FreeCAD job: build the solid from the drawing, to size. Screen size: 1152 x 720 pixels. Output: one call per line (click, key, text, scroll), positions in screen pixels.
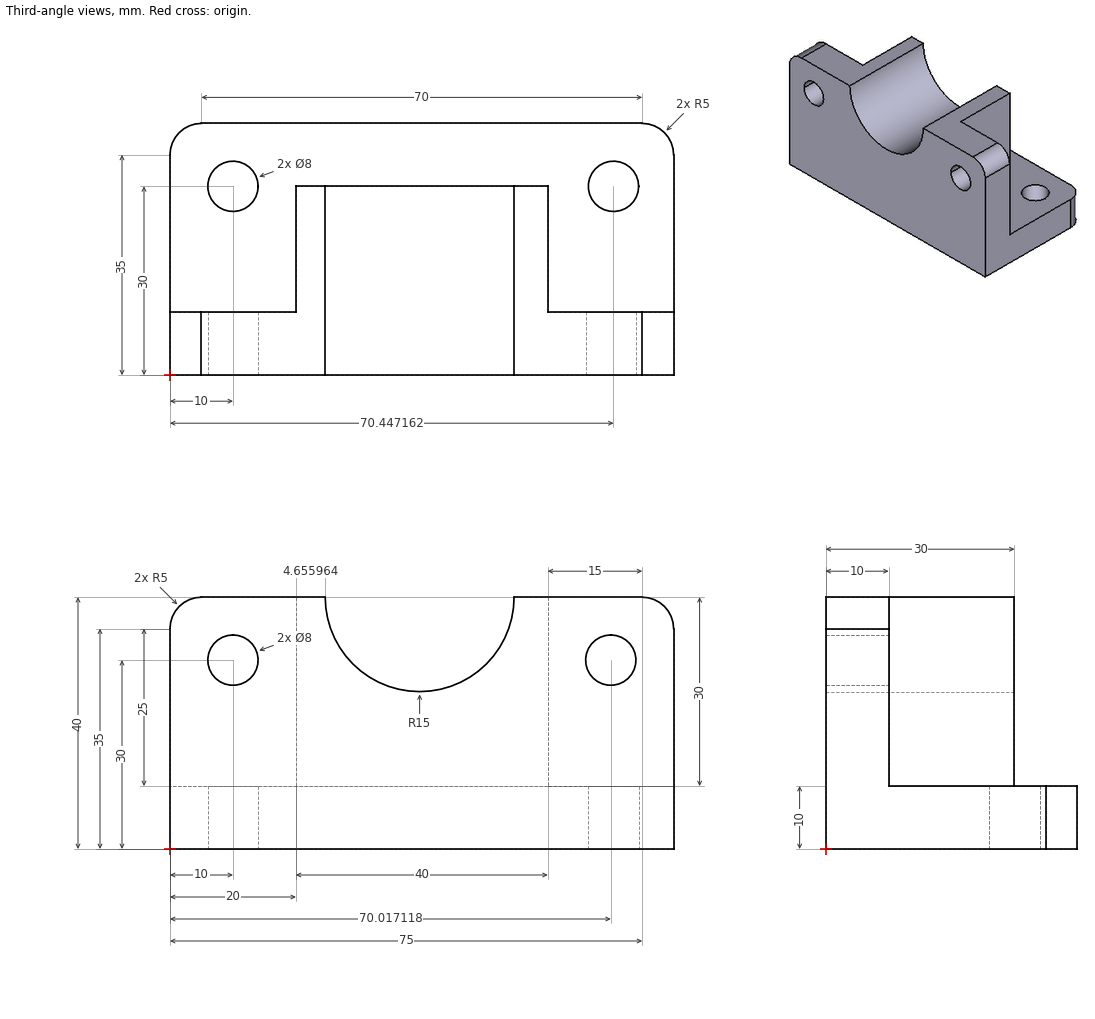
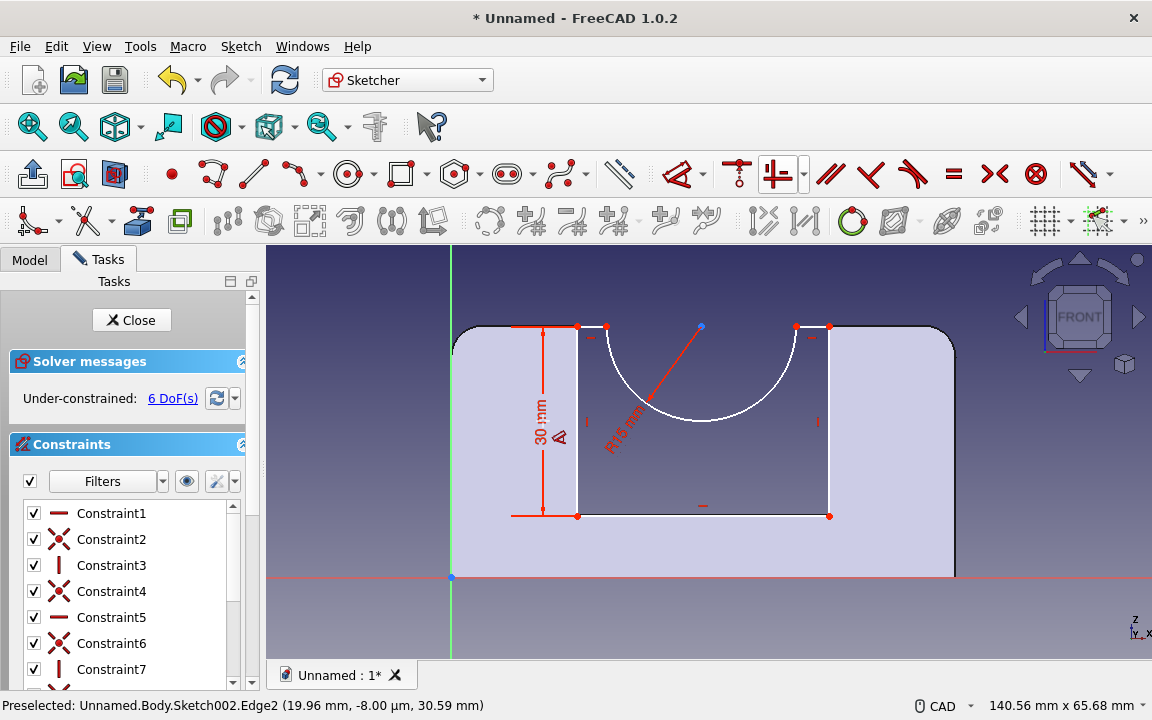
click(653, 516)
click(703, 550)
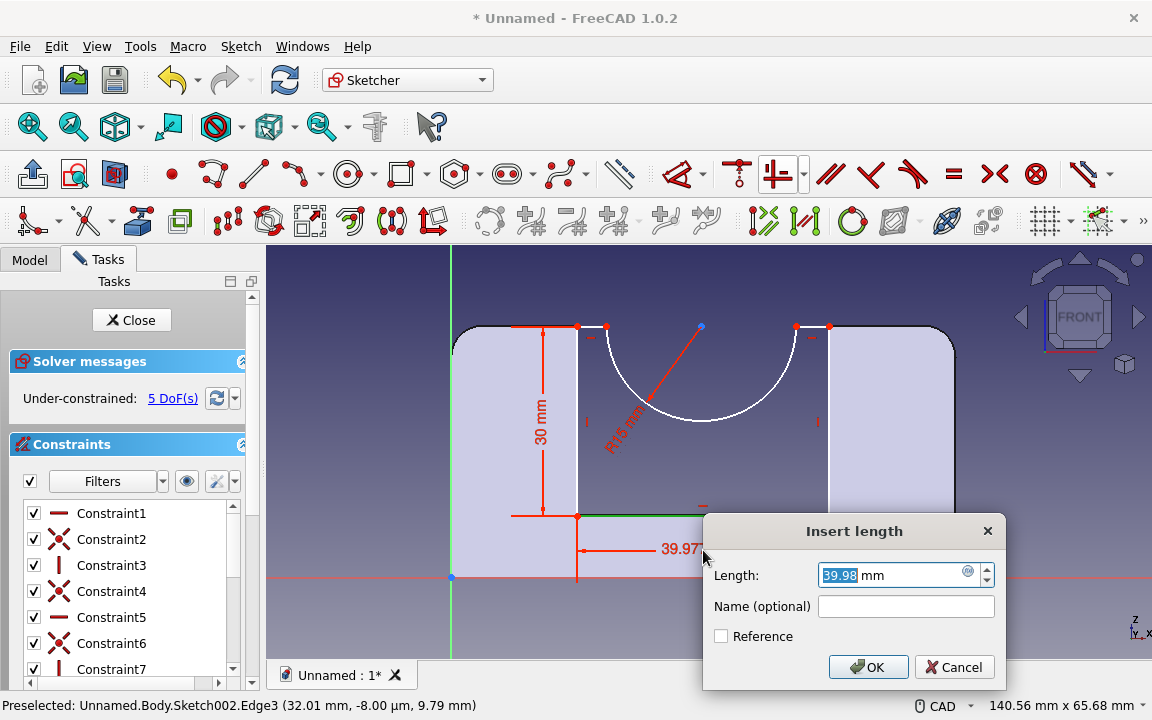
text(40)
key(Return)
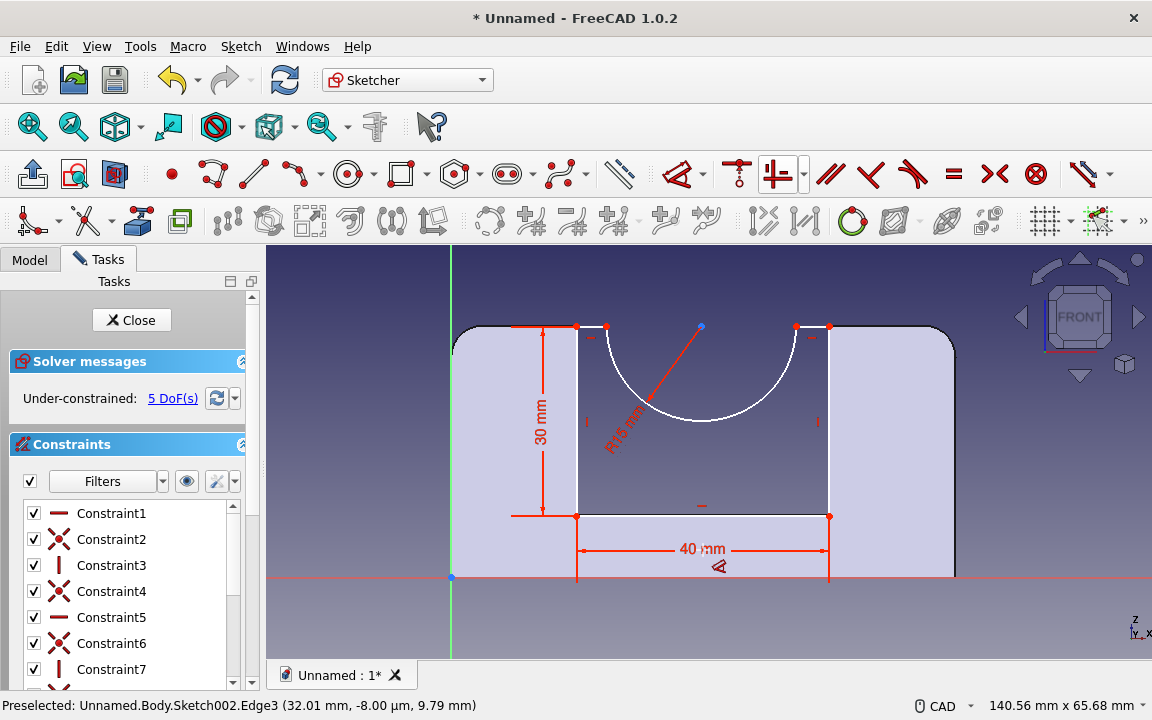
click(829, 459)
click(863, 422)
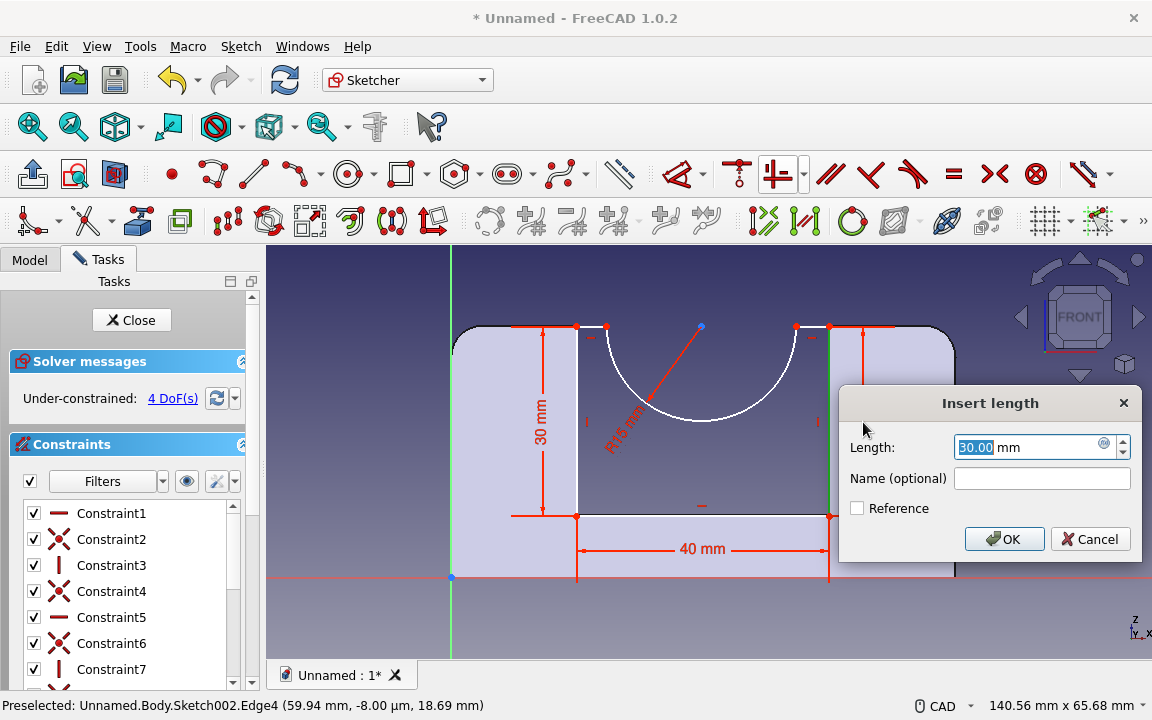
text(30)
key(Return)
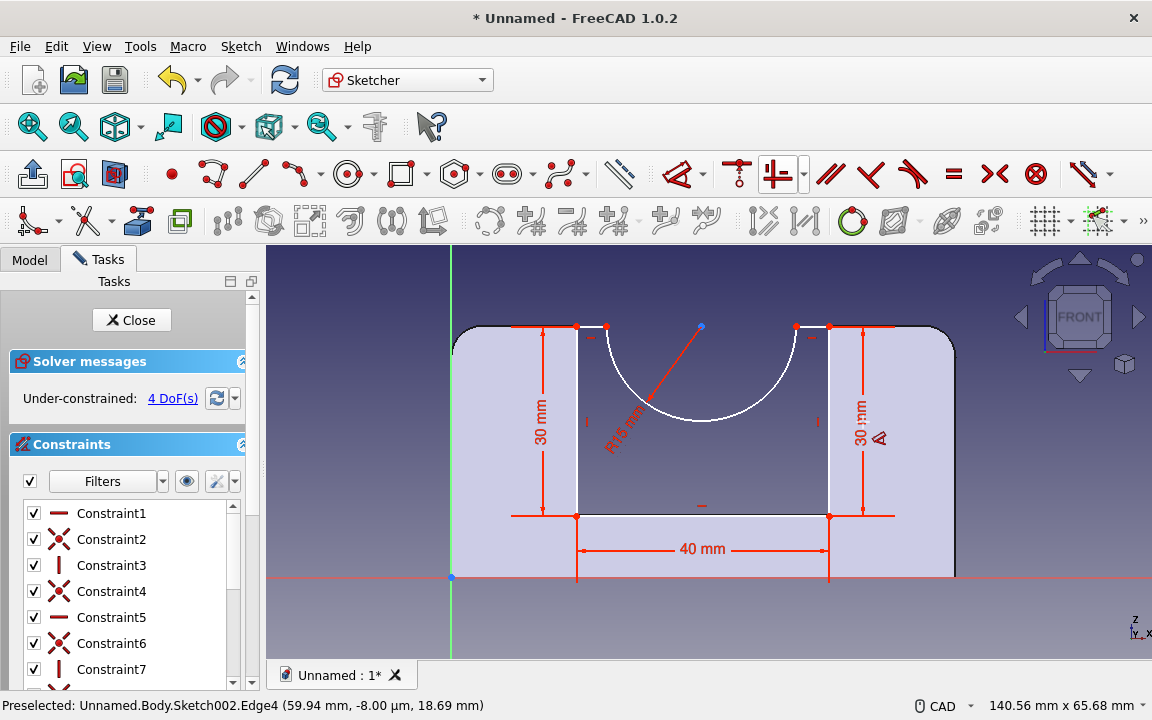
click(607, 327)
click(417, 452)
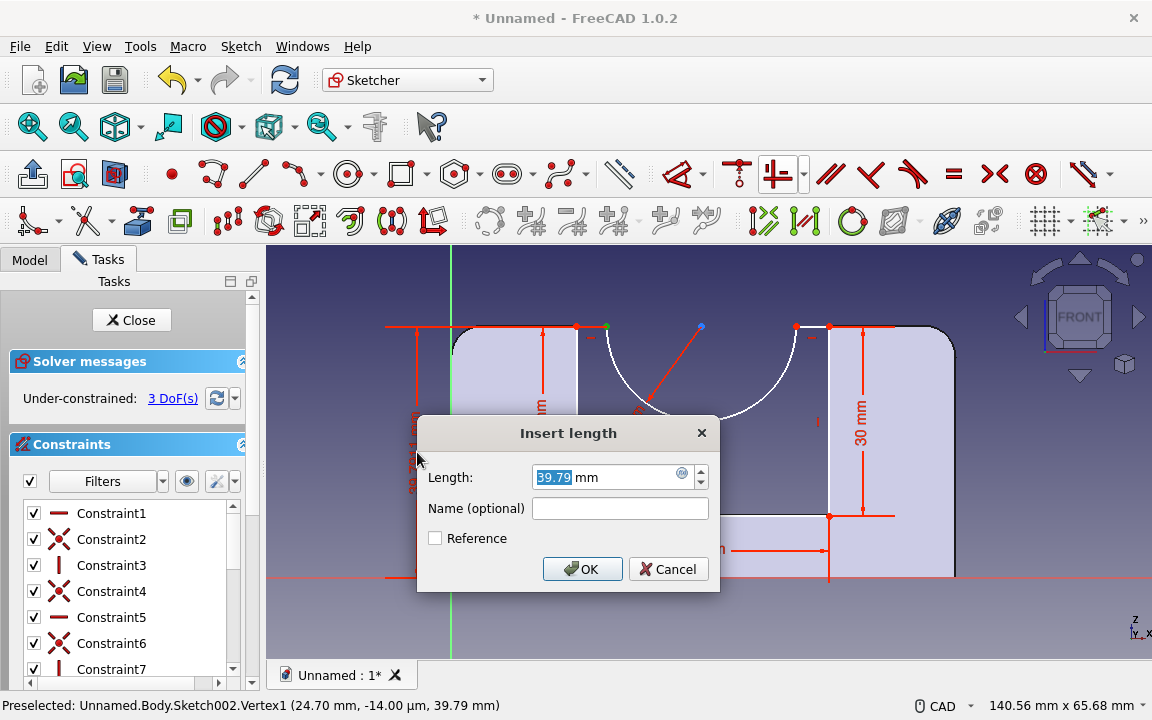
text(40)
key(Return)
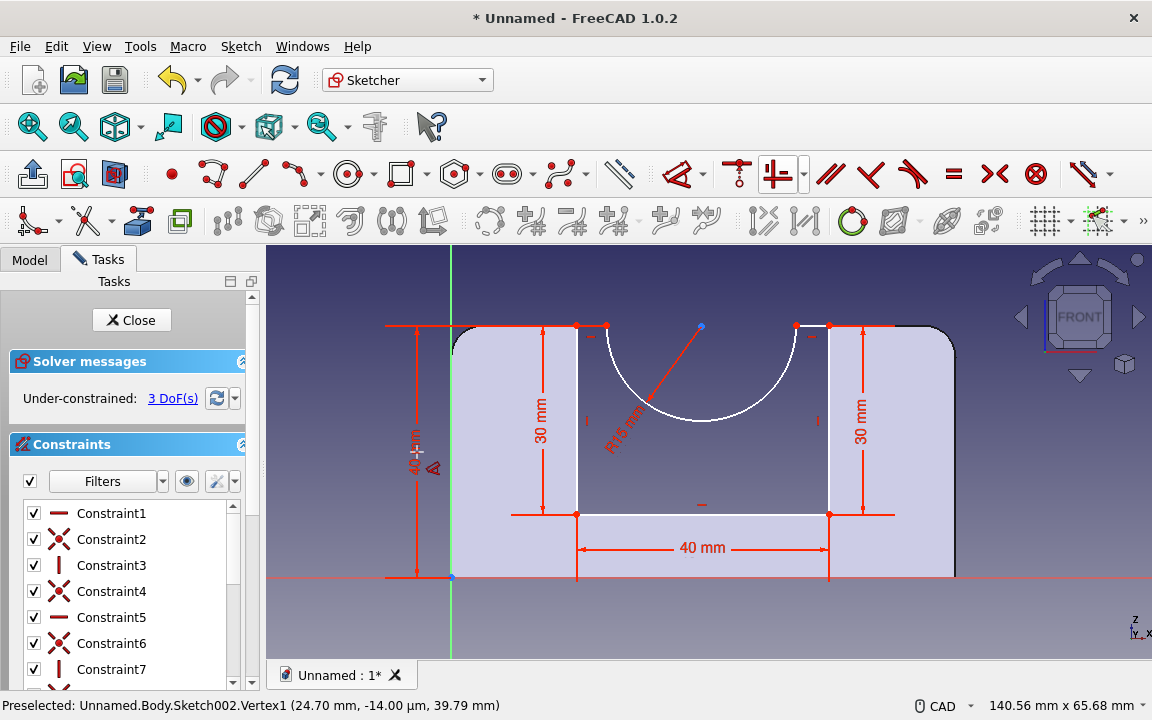
click(577, 326)
click(514, 612)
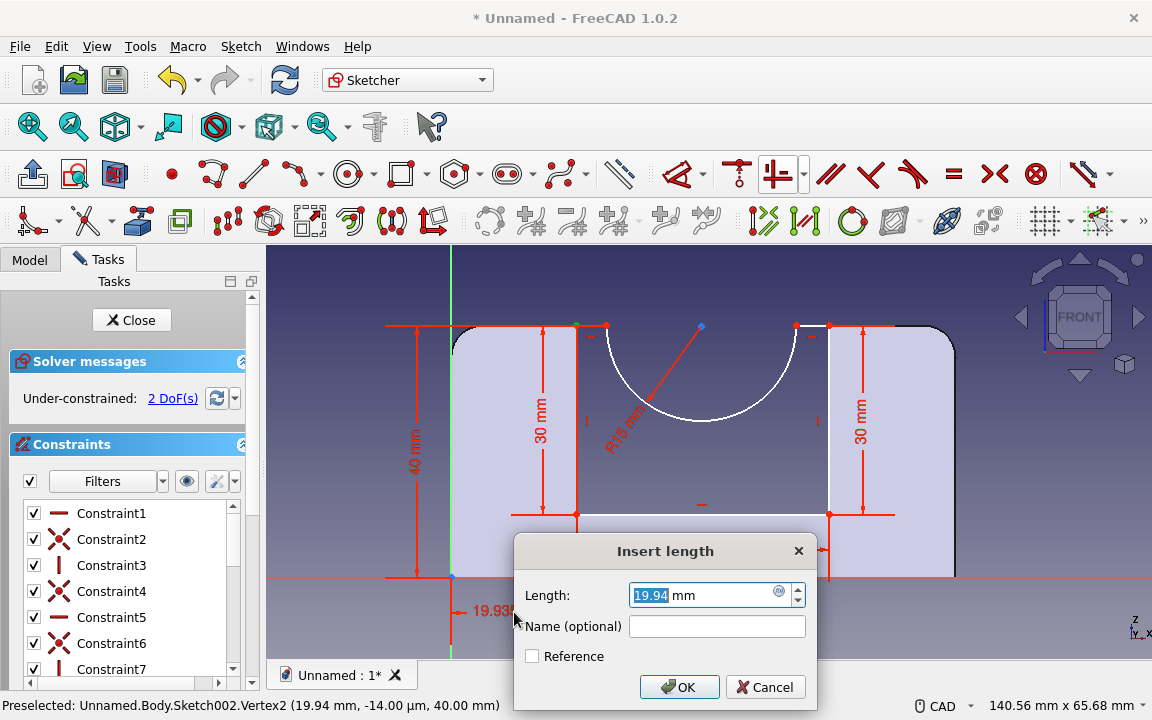
text(20)
key(Return)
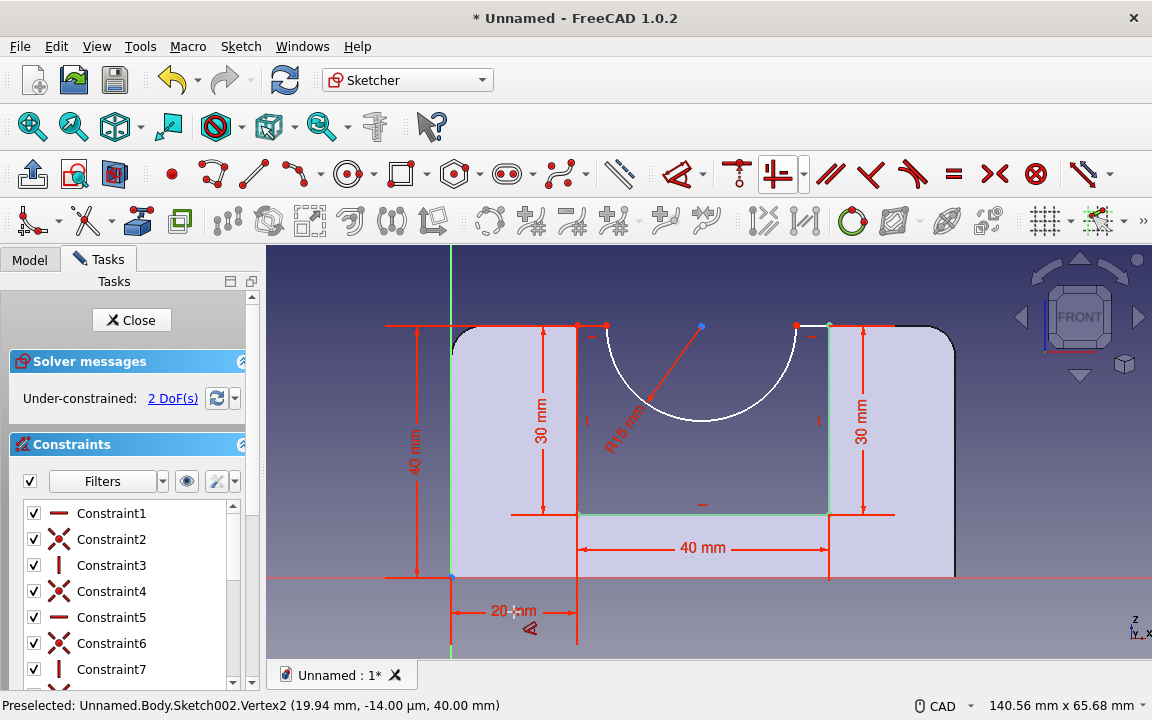
click(701, 327)
click(417, 394)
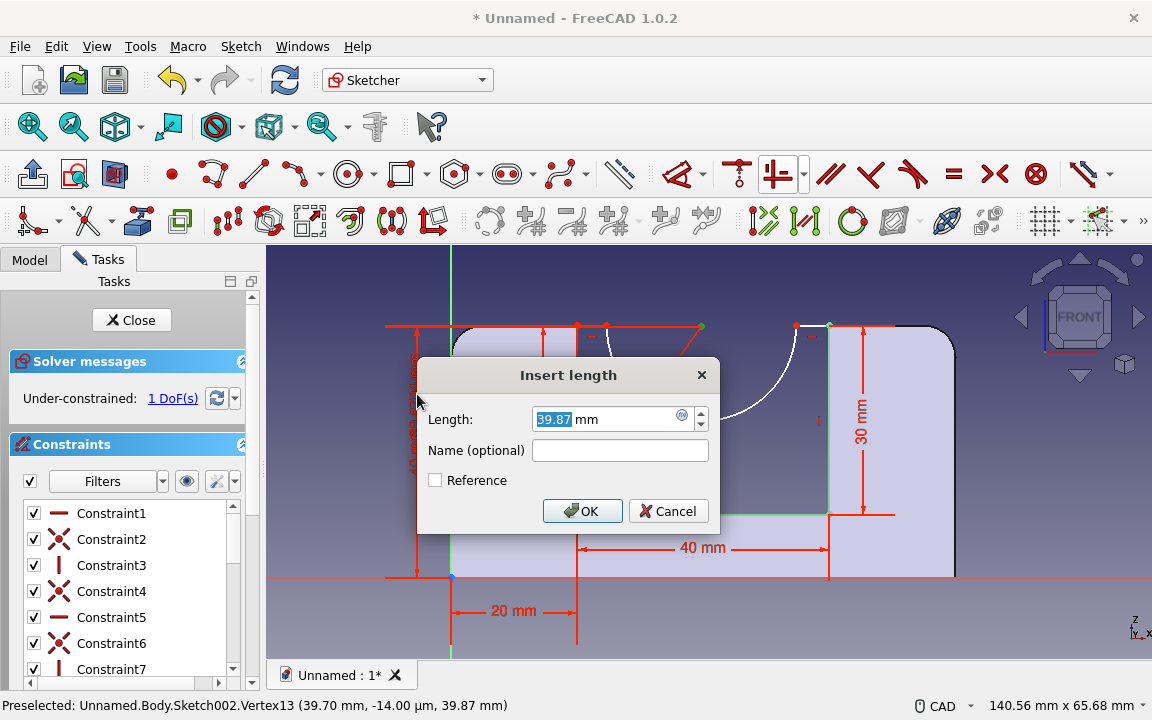
text(40)
key(Return)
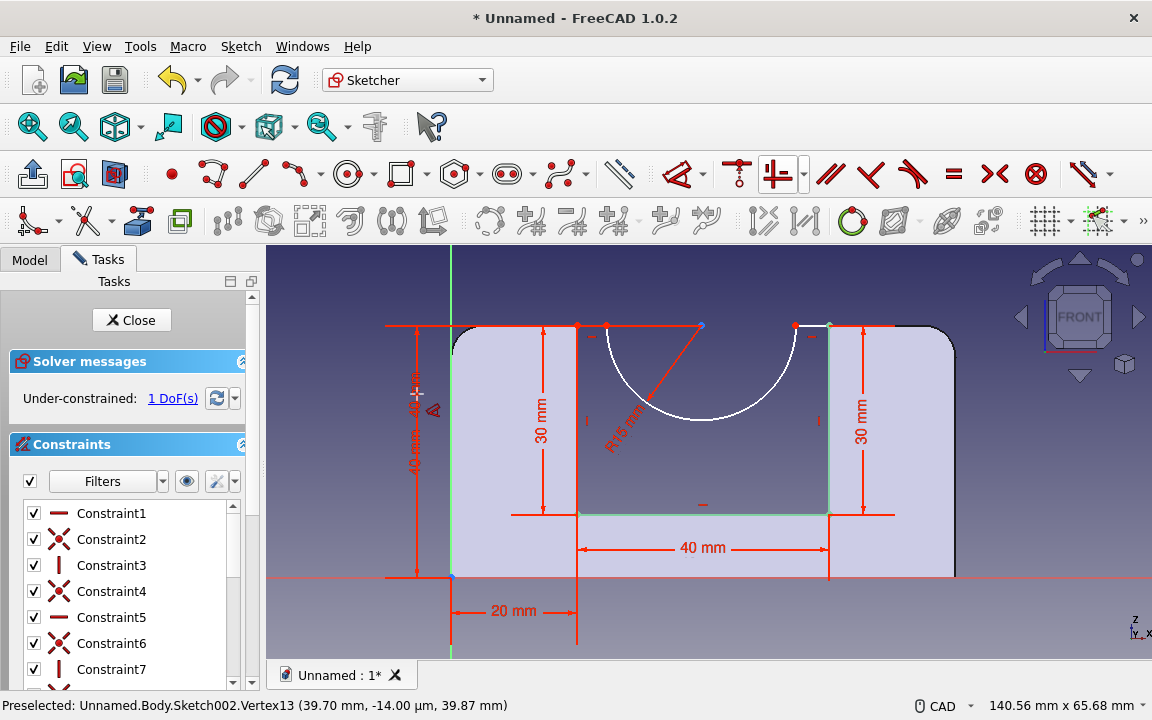
scroll(595, 326, up, 2)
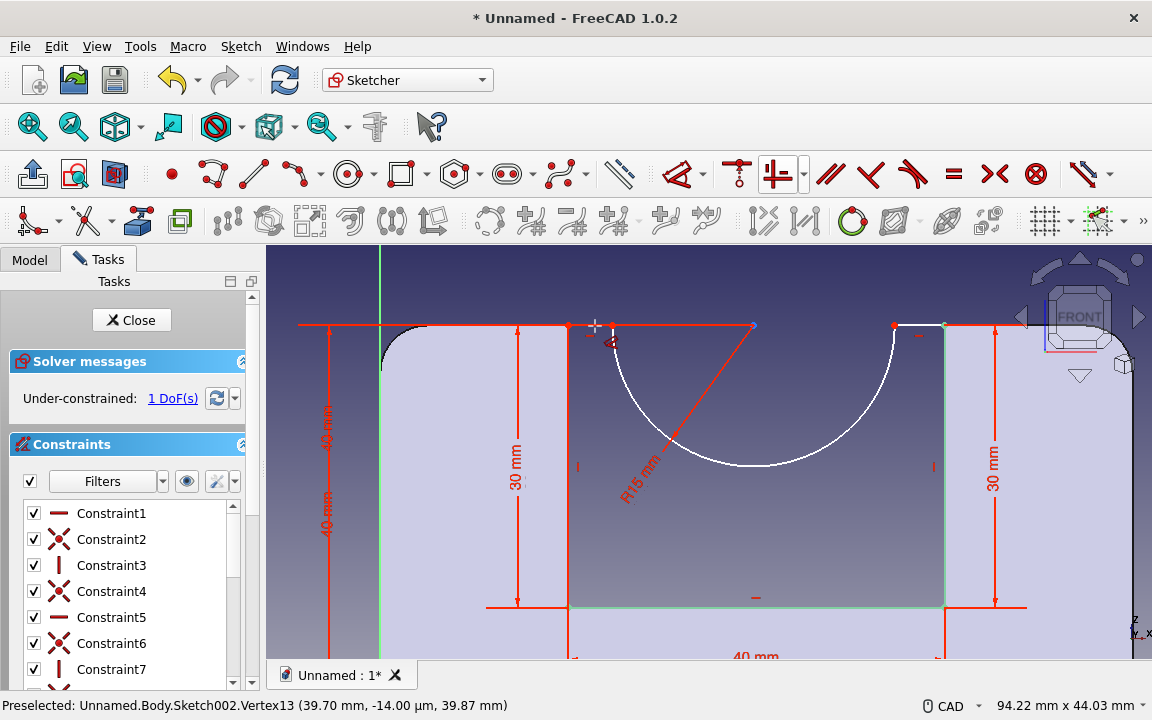
click(595, 325)
click(590, 291)